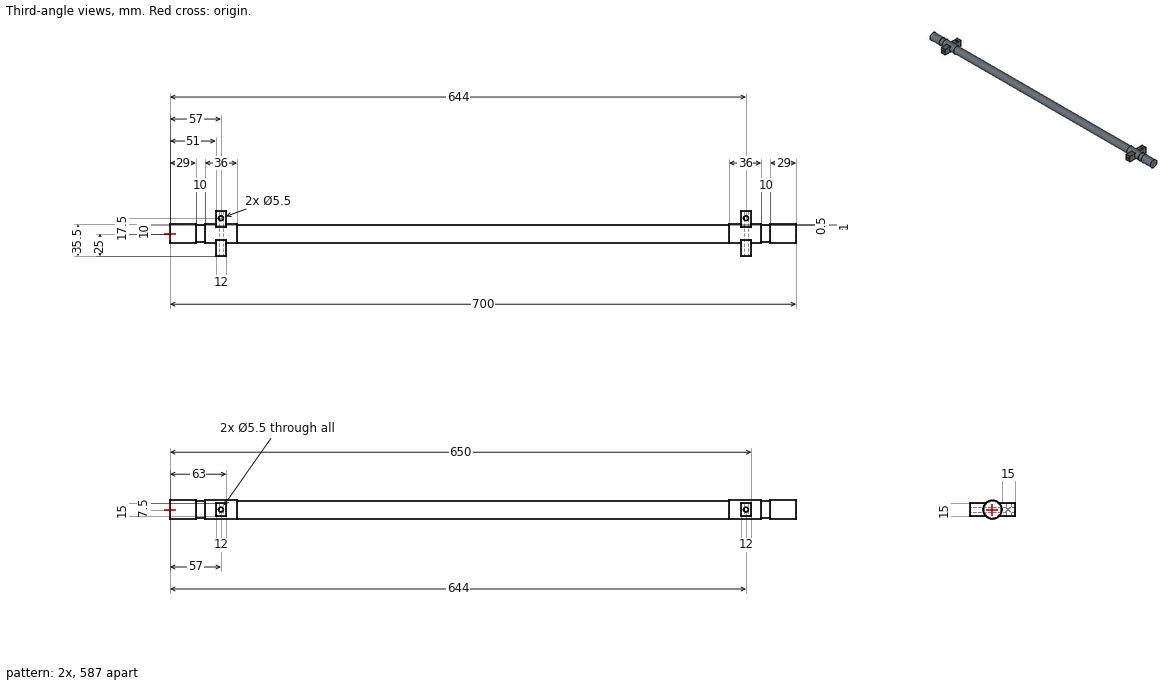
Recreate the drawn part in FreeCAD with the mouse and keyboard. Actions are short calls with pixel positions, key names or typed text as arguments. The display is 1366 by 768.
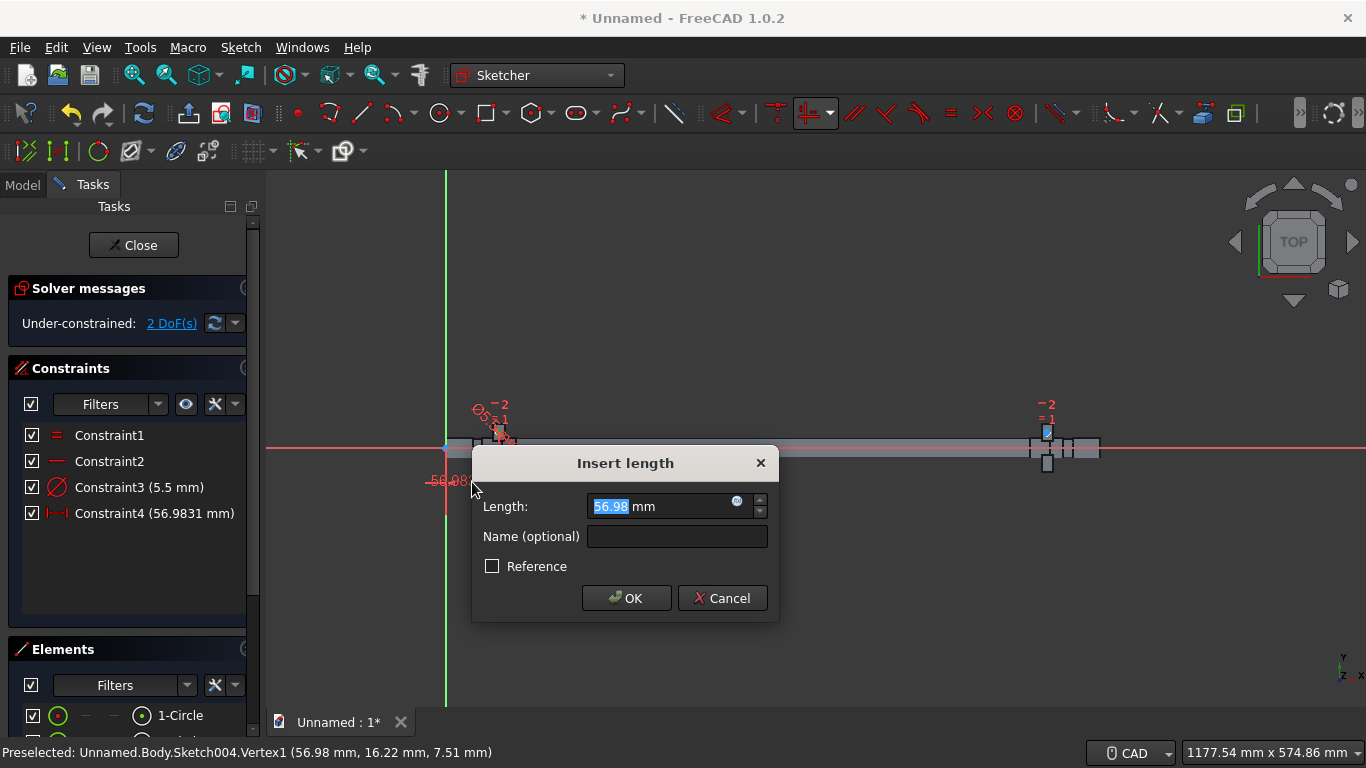
text(57)
key(Return)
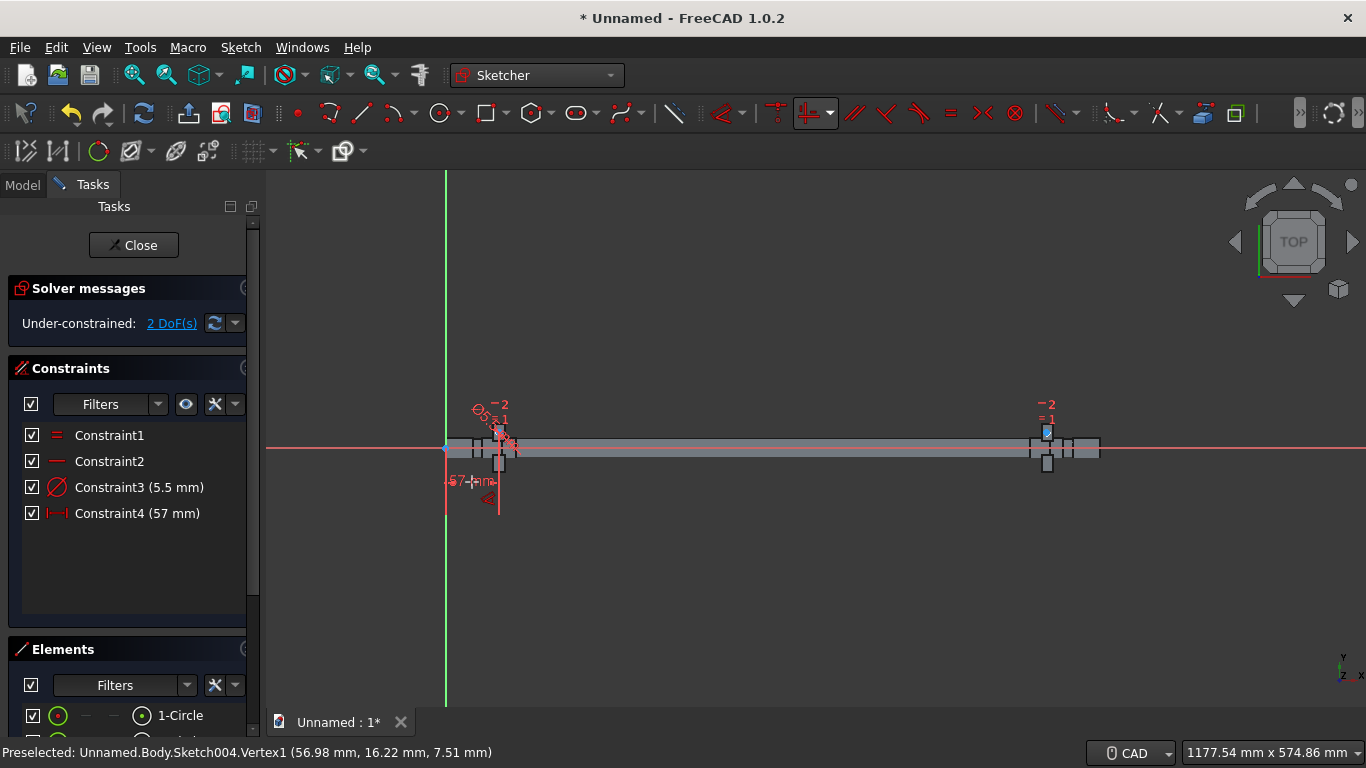
click(1047, 433)
click(746, 482)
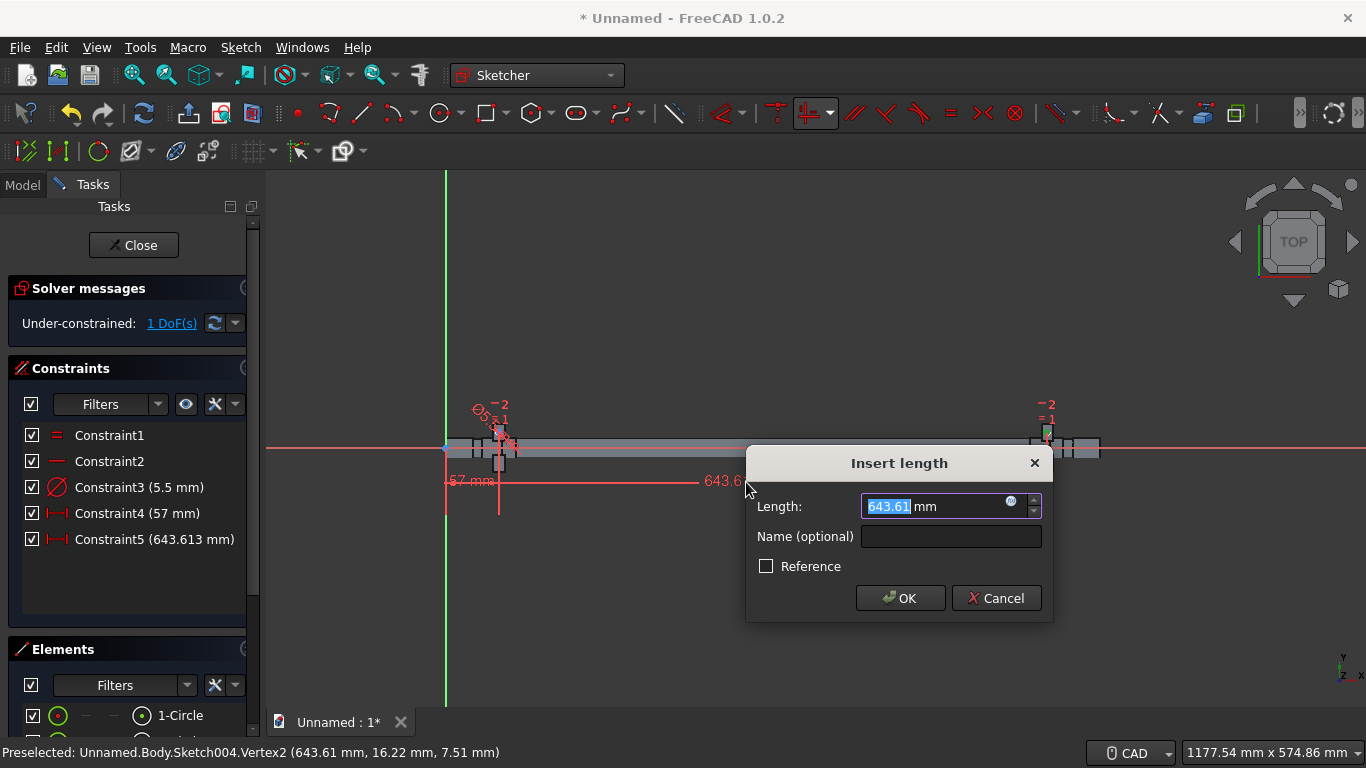
text(644)
key(Return)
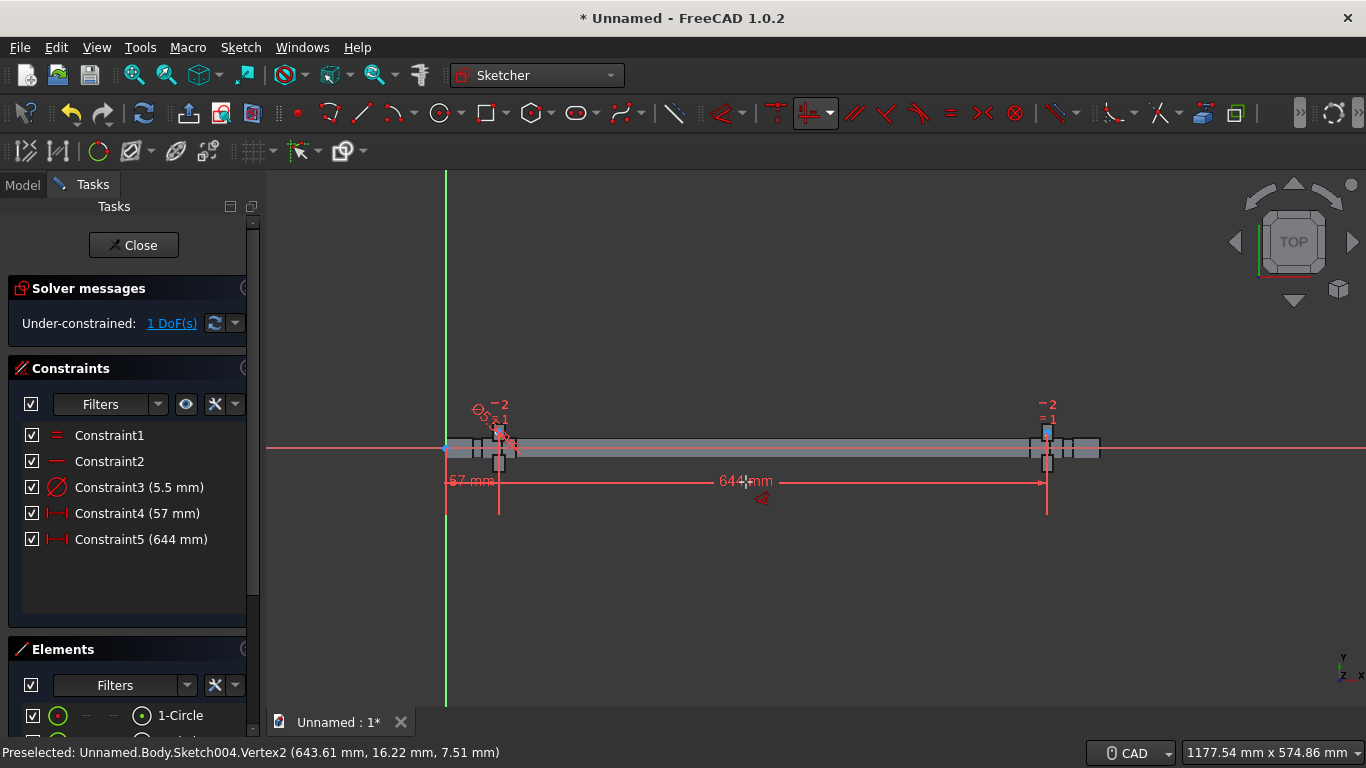
scroll(499, 433, up, 5)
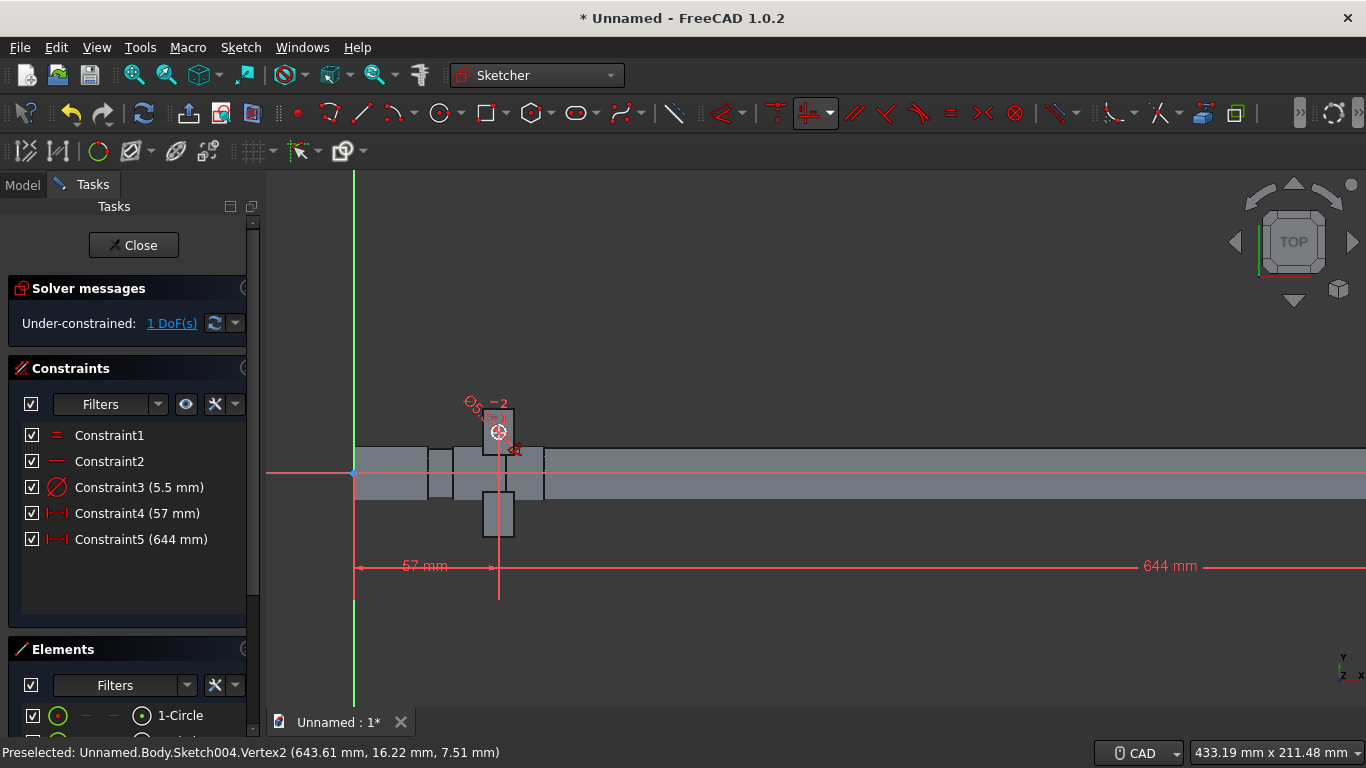
click(499, 432)
click(320, 453)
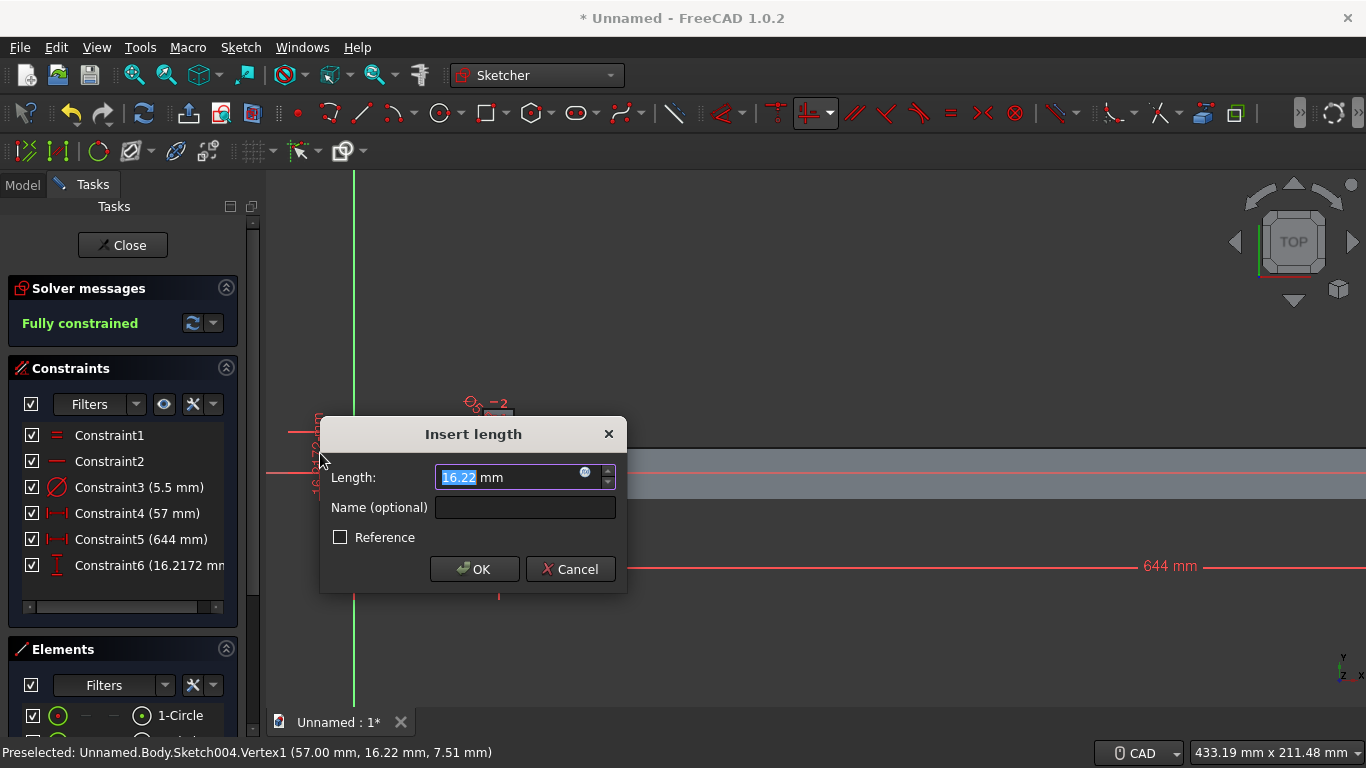
text(17.5)
key(Return)
key(Escape)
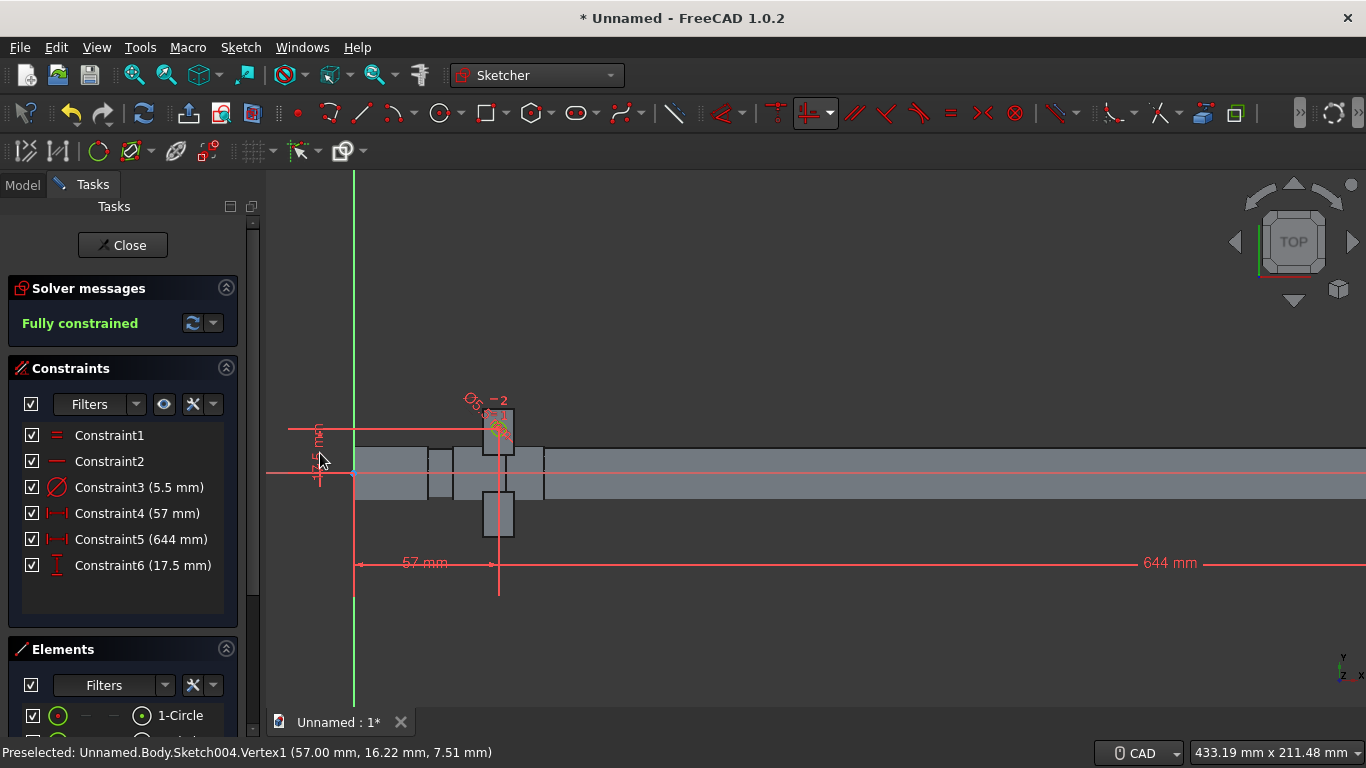
click(123, 245)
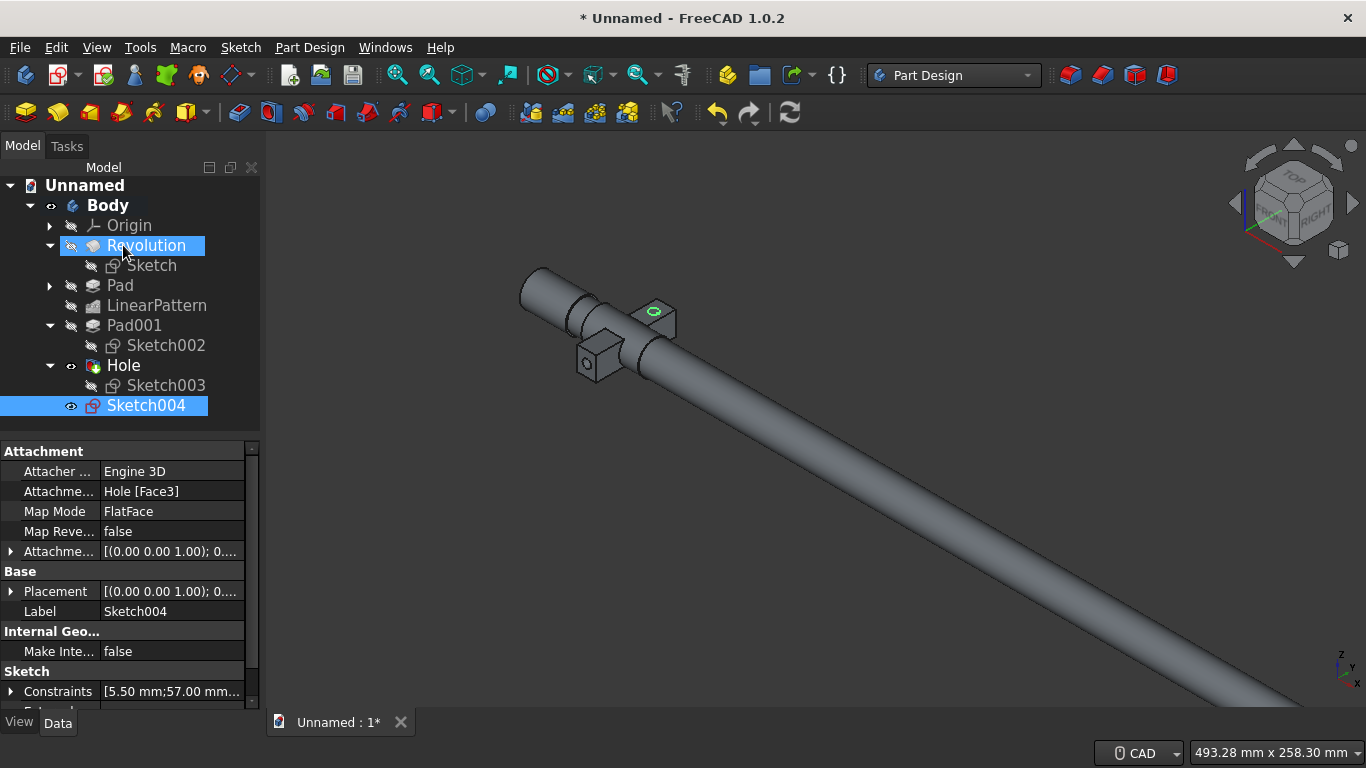
click(240, 112)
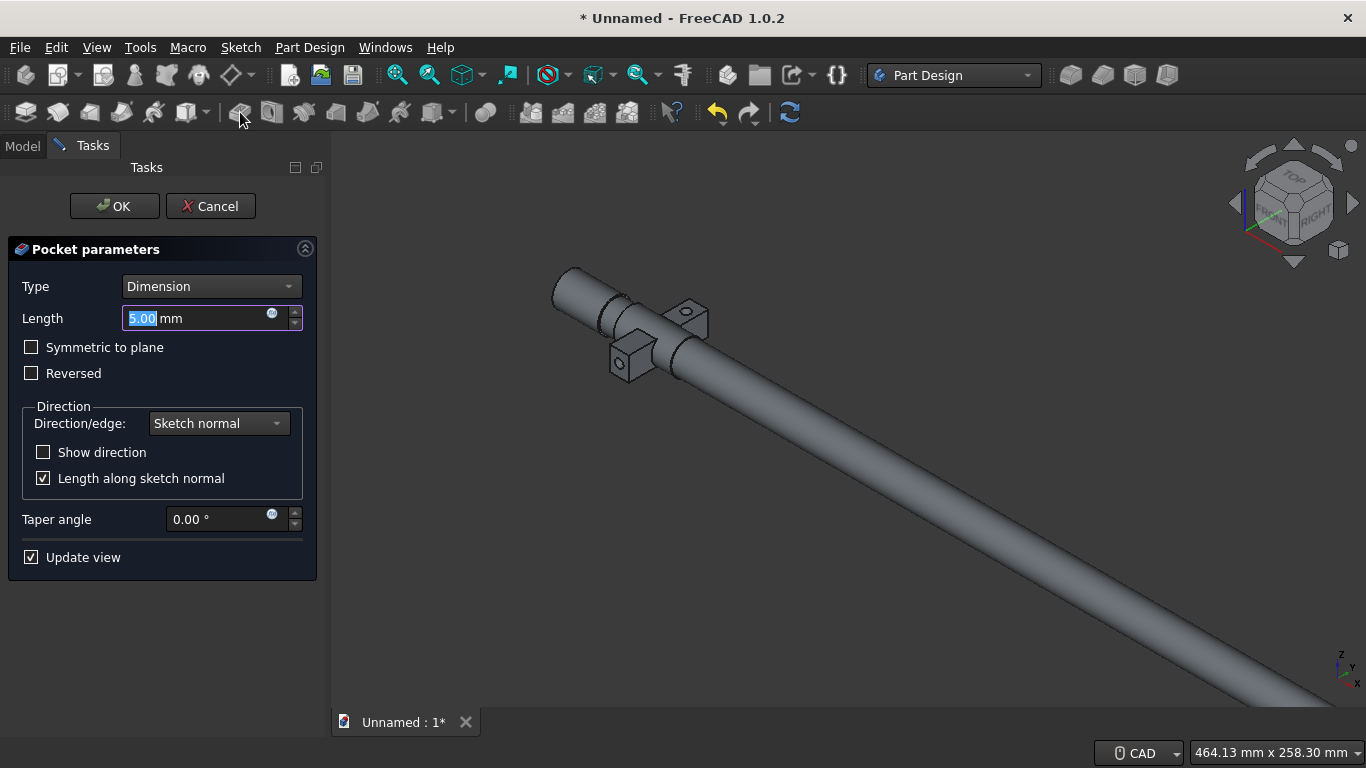
click(212, 286)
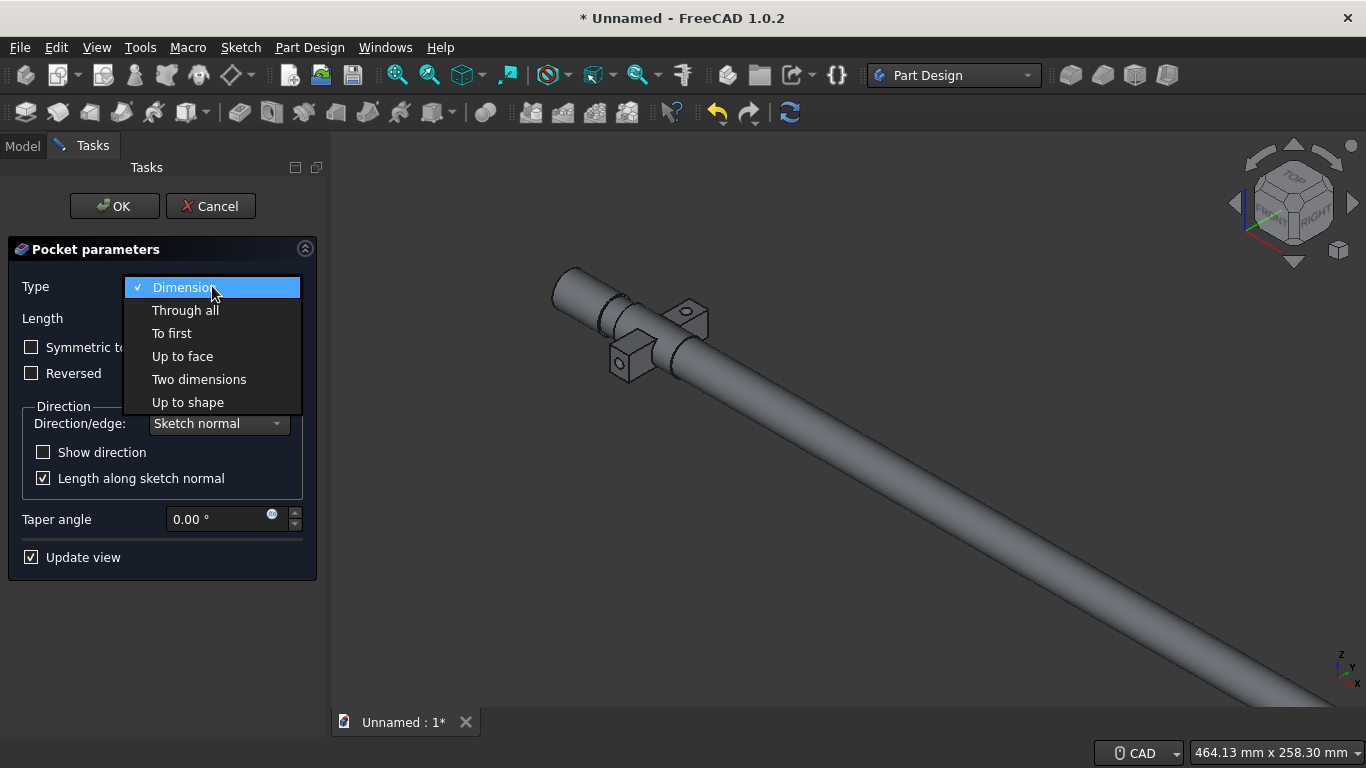
click(212, 310)